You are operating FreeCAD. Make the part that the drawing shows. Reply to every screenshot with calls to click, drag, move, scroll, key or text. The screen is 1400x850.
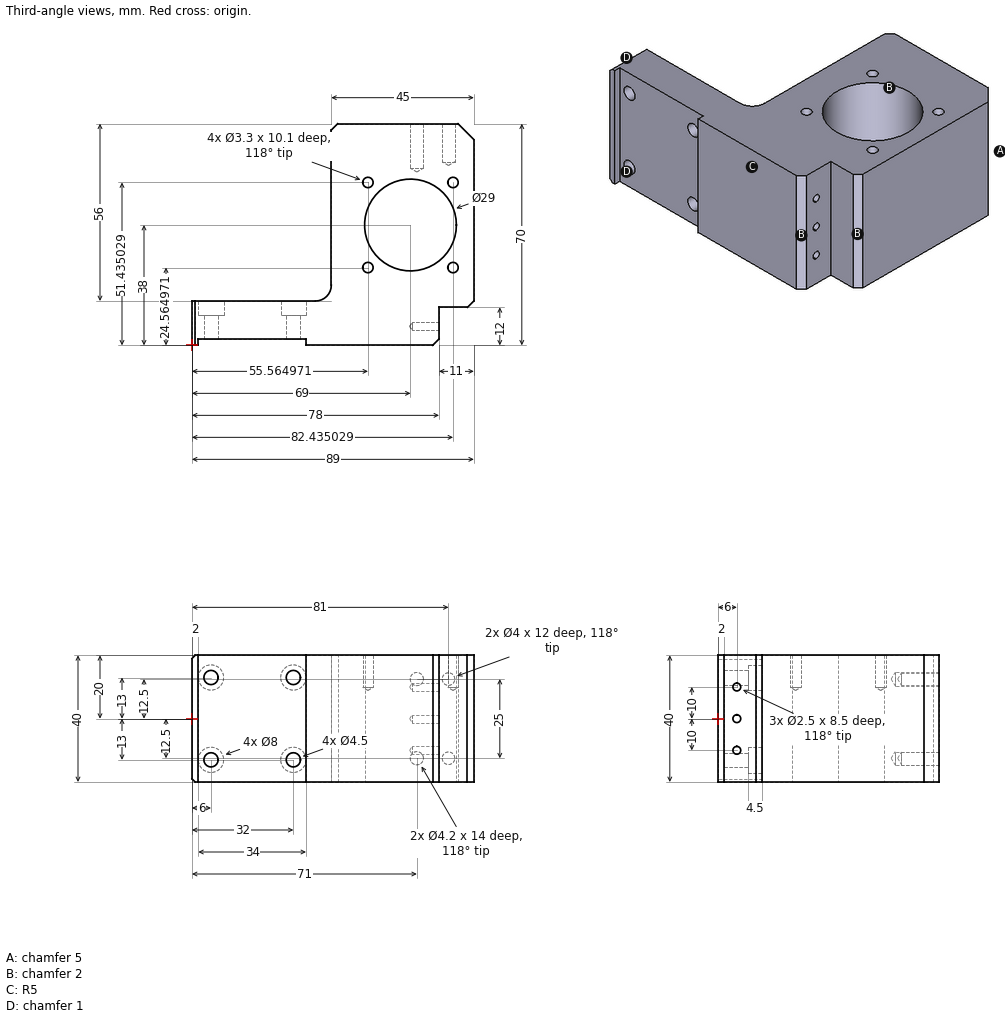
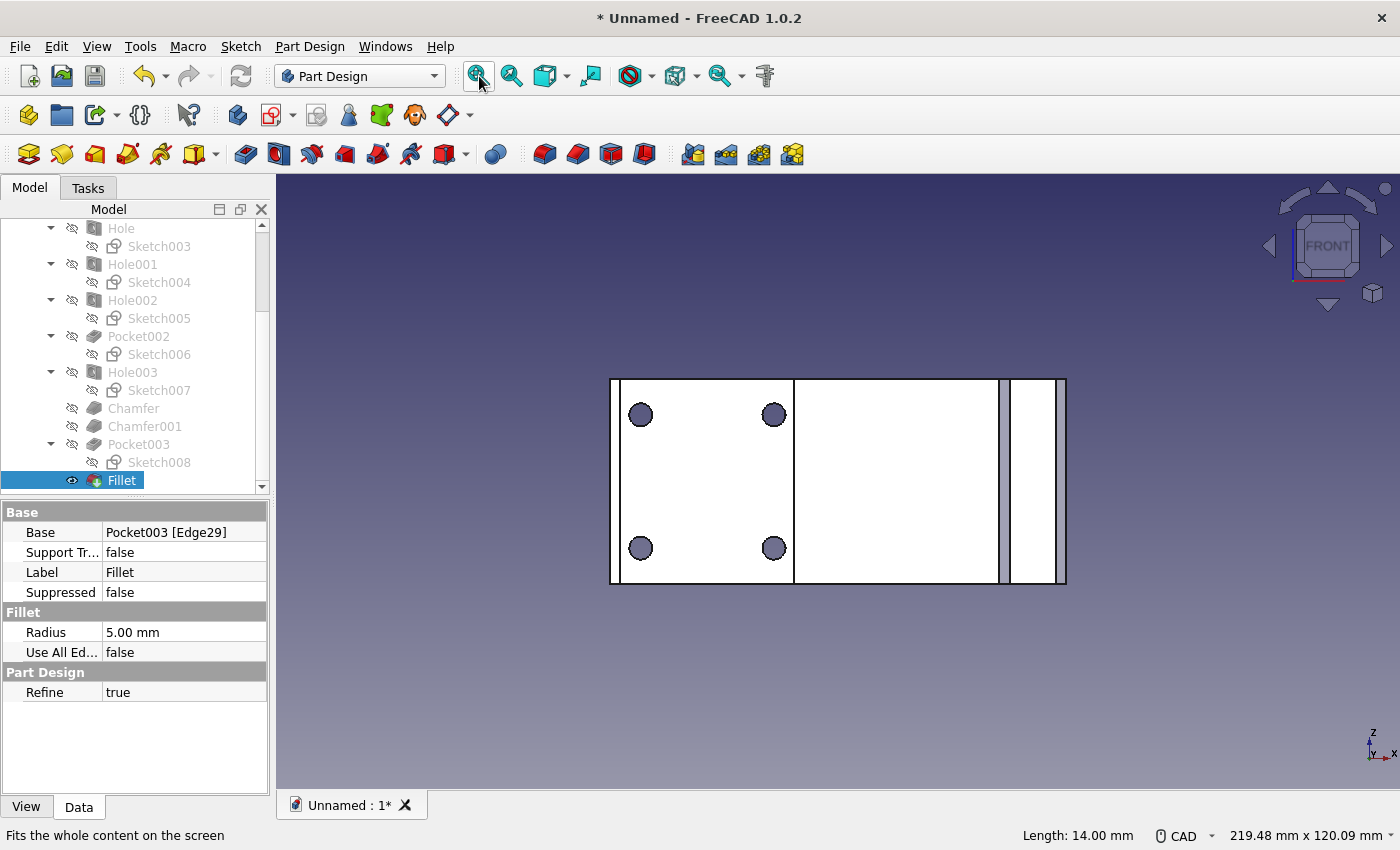
key(3)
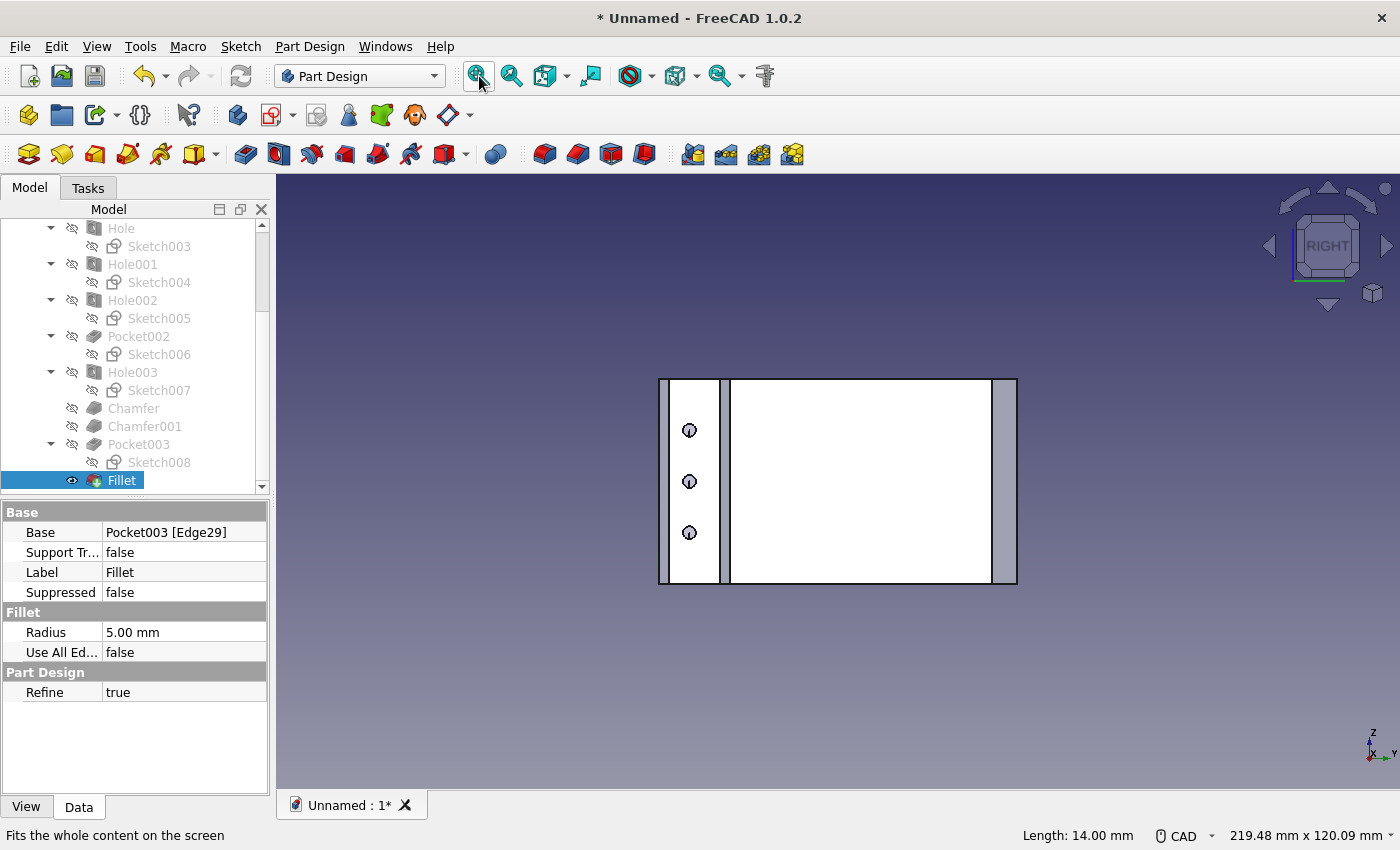
click(479, 76)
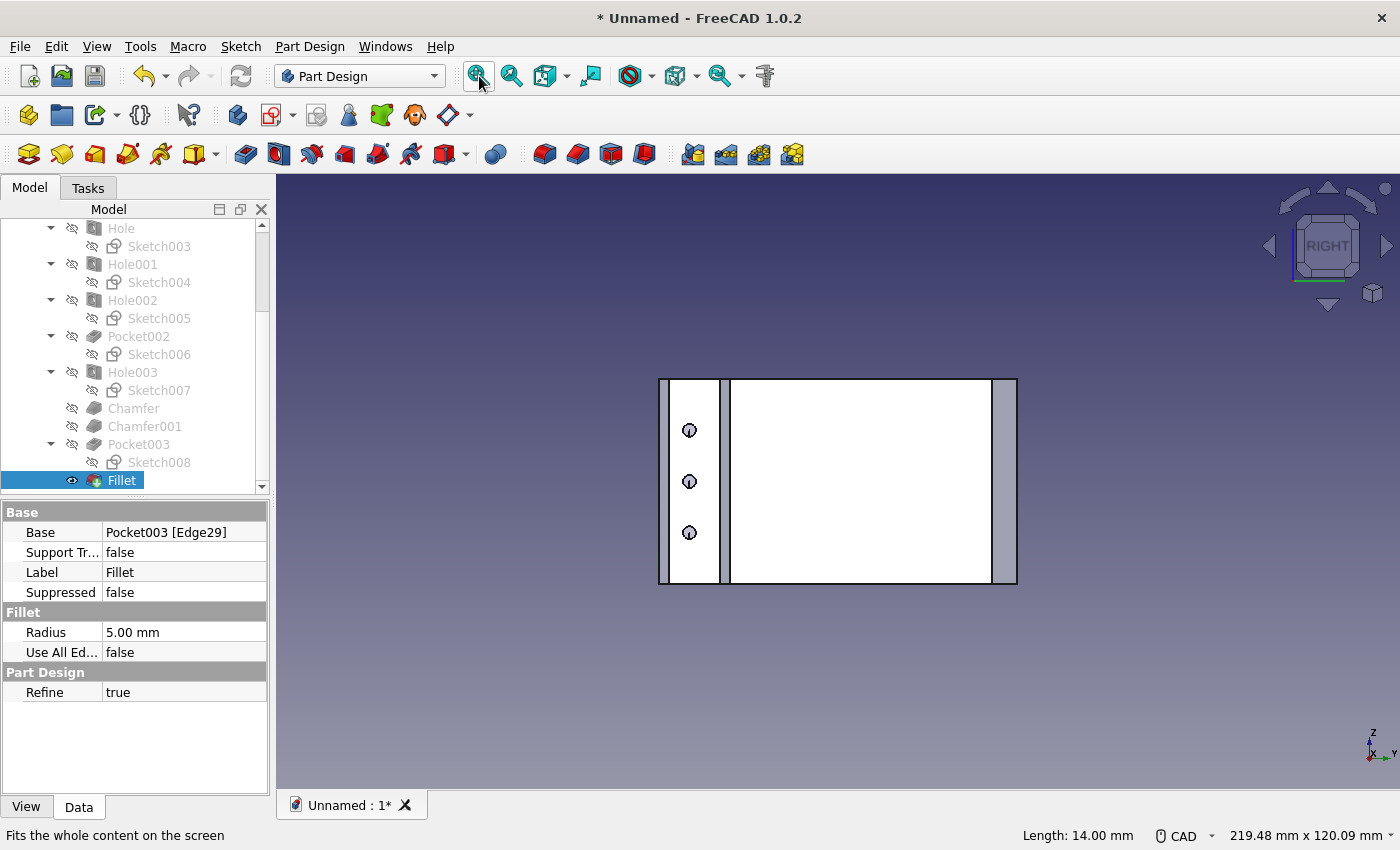
key(5)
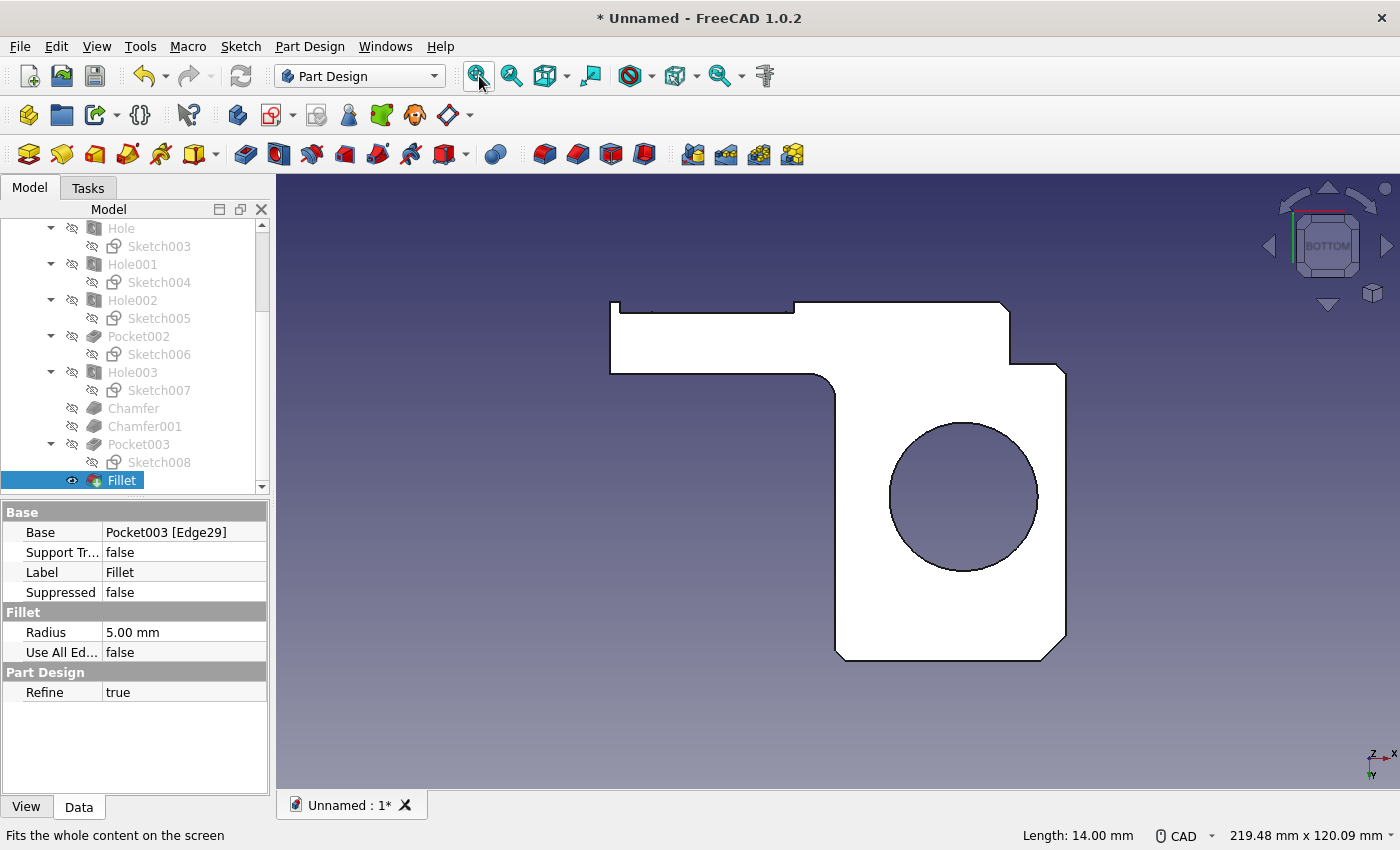
click(610, 337, ctrl)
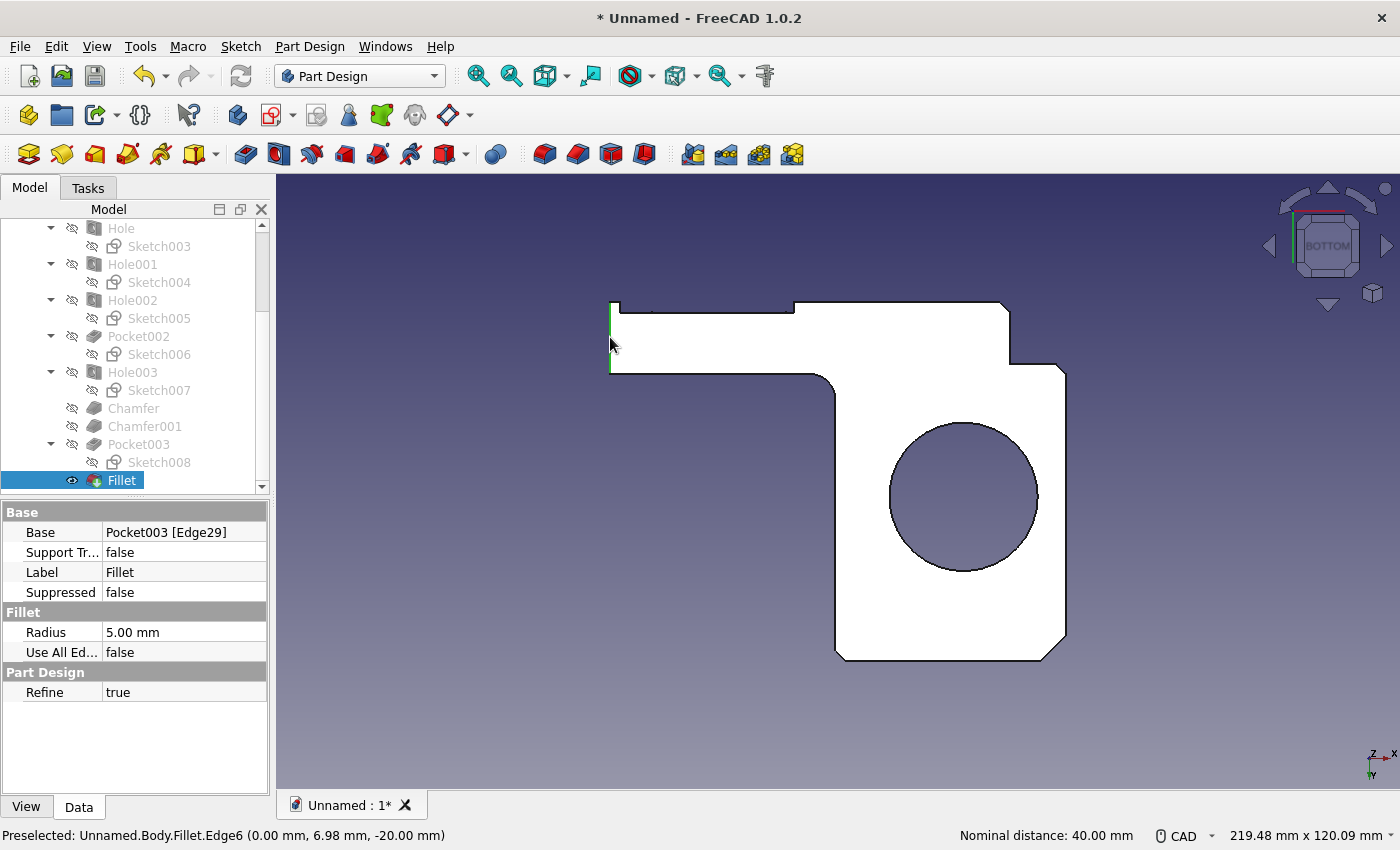
click(578, 154)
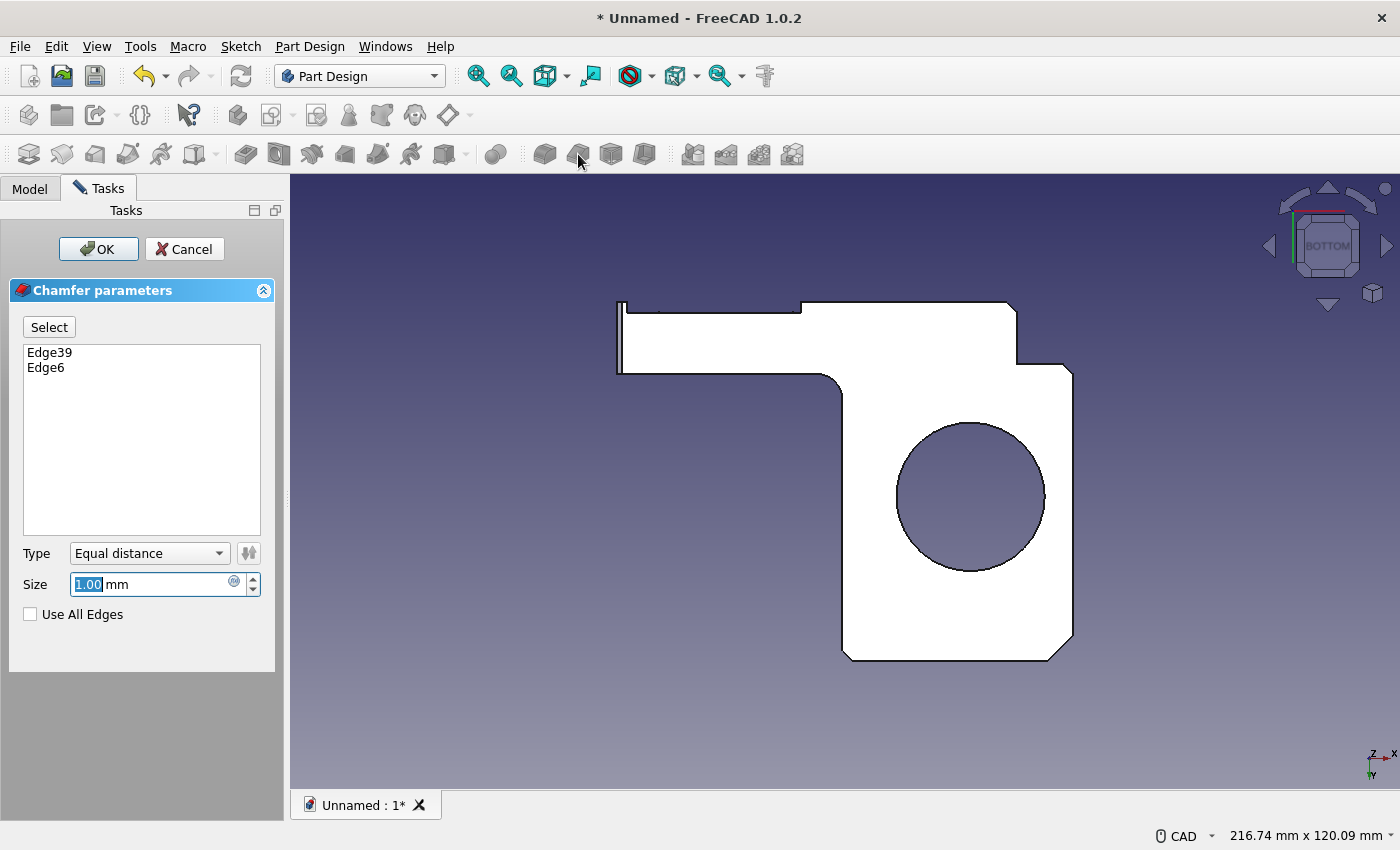
text(1)
key(Tab)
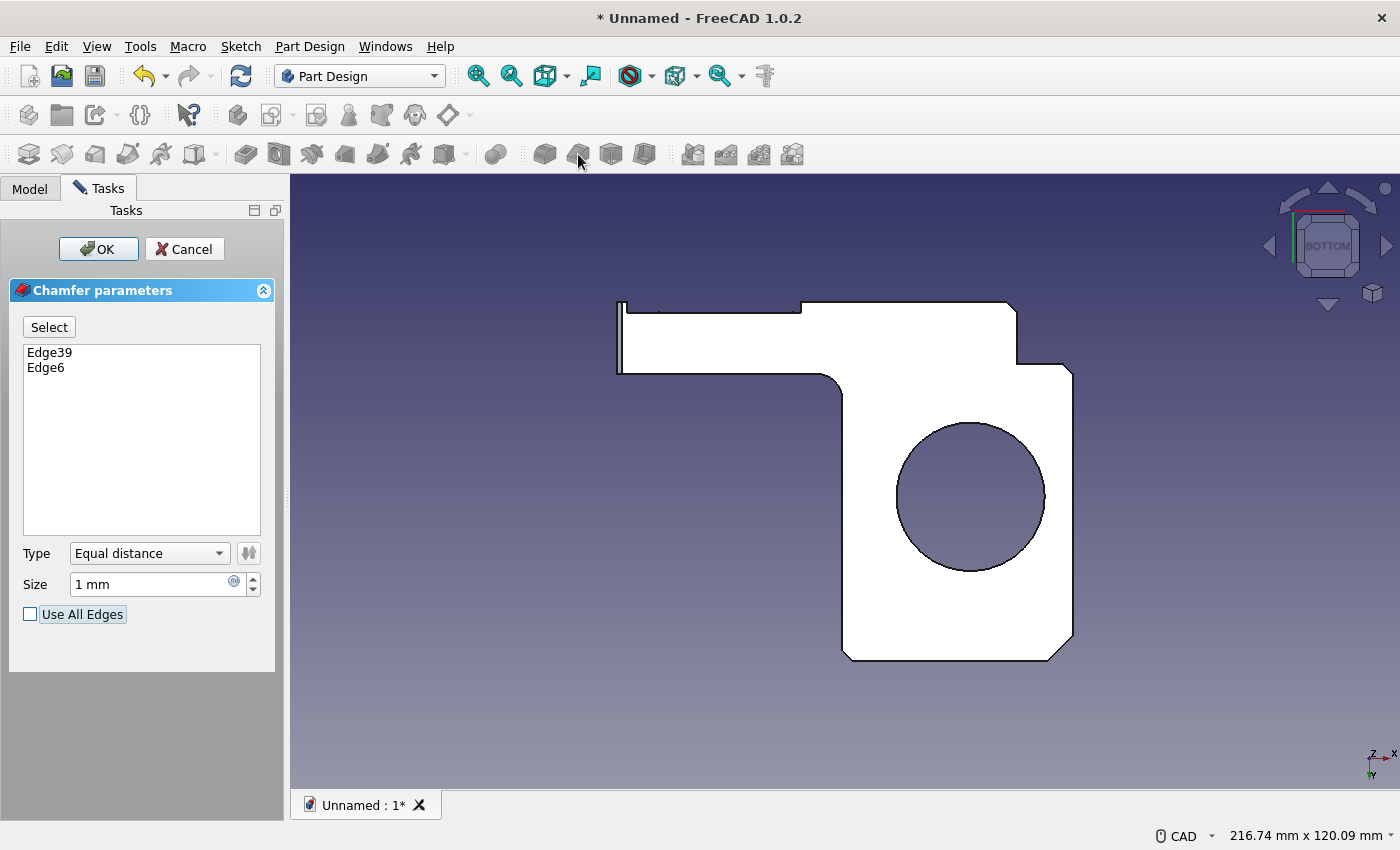
click(99, 249)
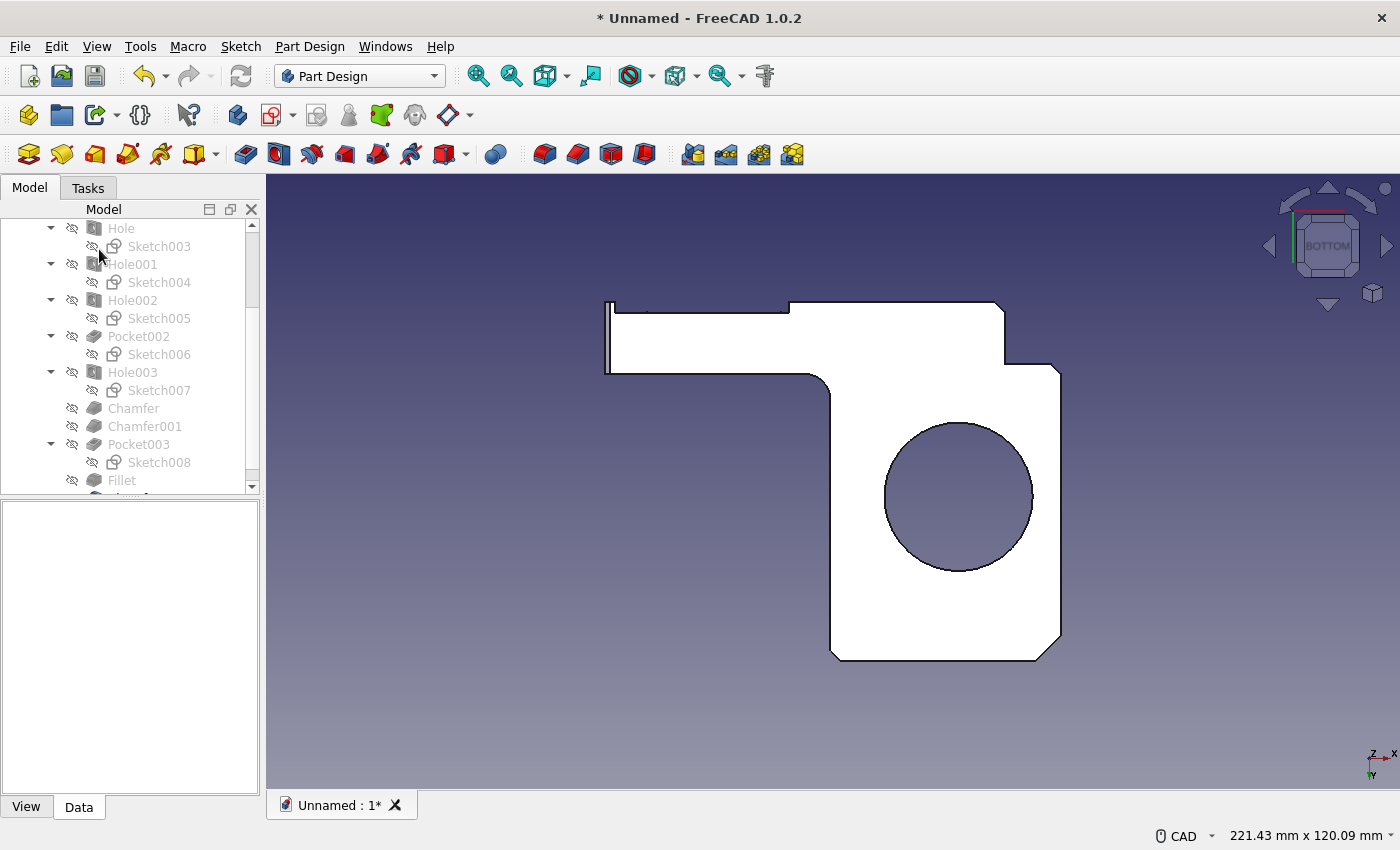
key(0)